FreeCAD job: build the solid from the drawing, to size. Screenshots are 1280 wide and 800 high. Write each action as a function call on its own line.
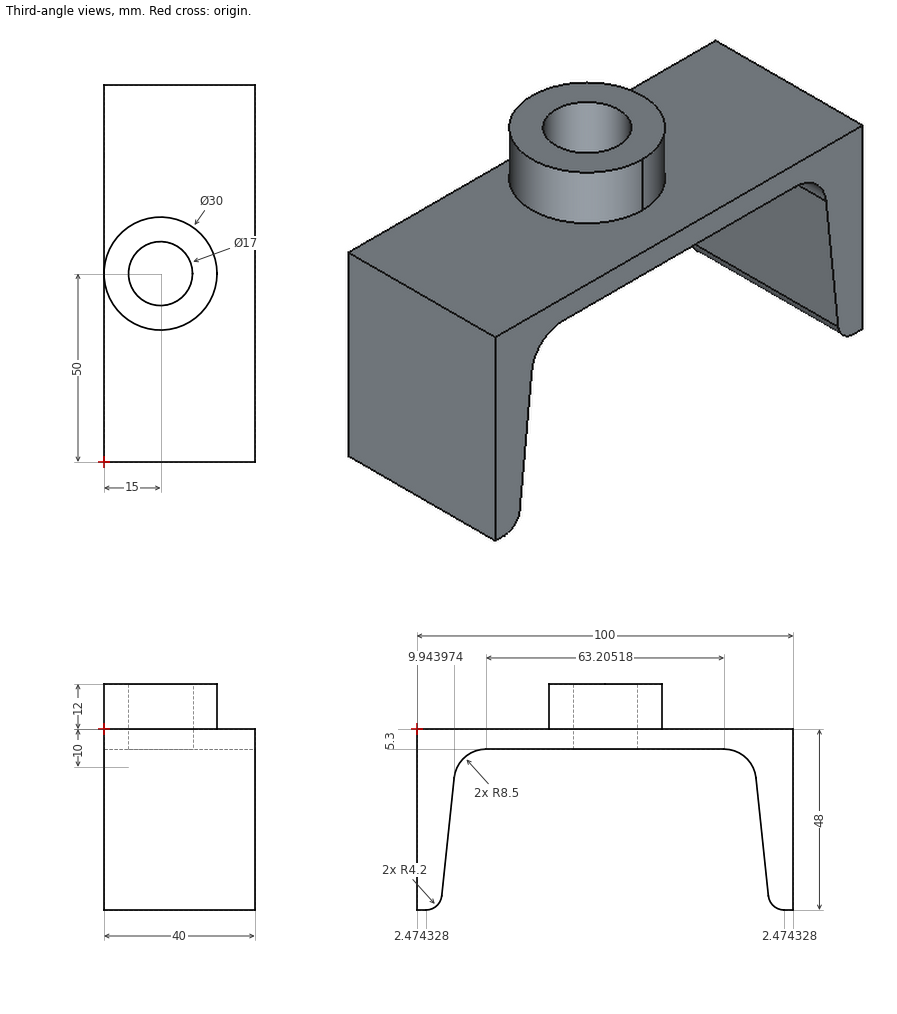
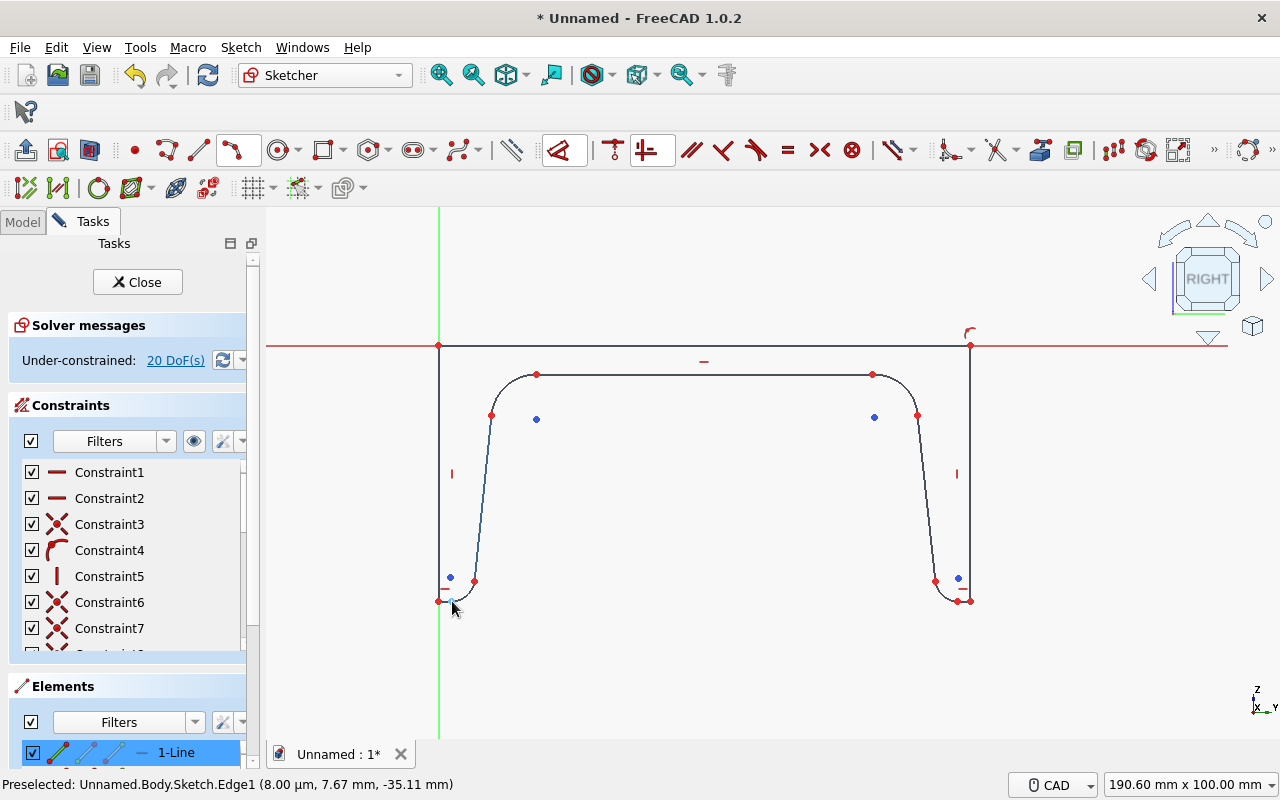
click(517, 379)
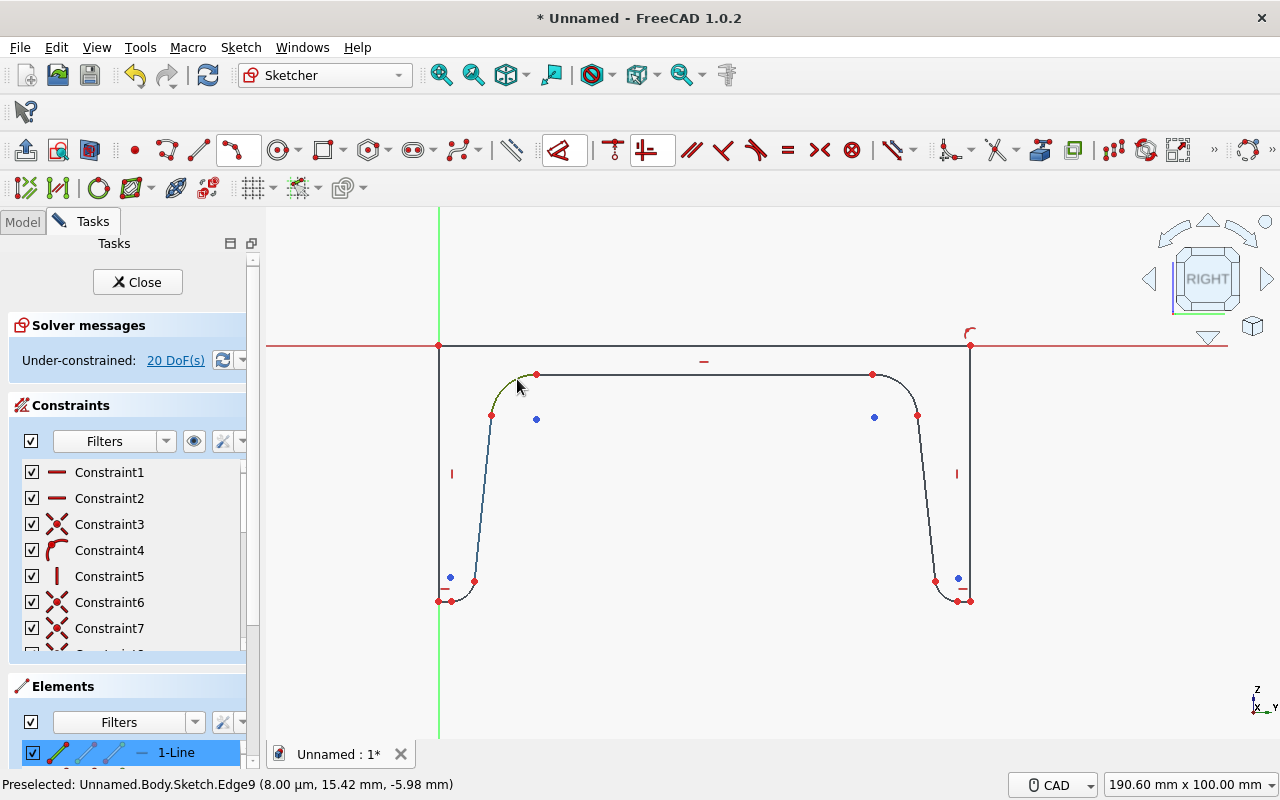
click(756, 150)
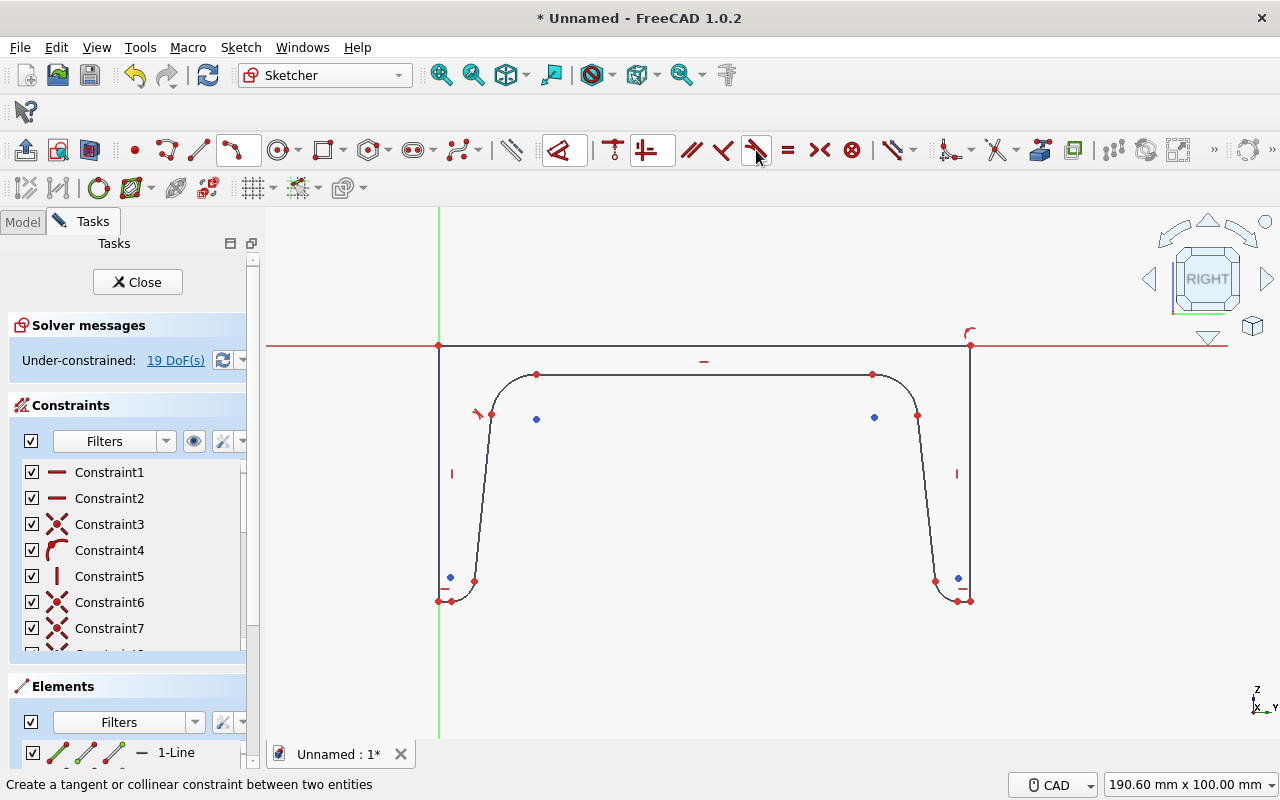
click(480, 532)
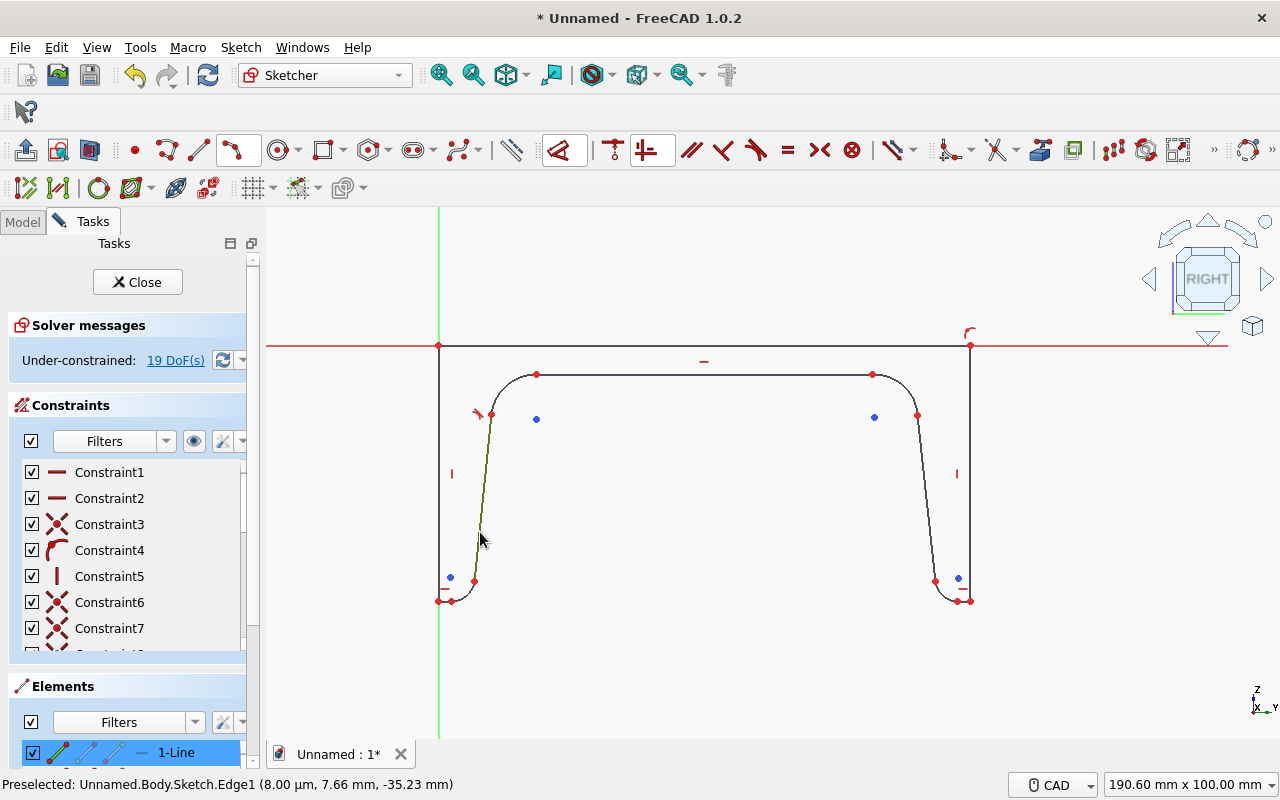
scroll(461, 599, up, 2)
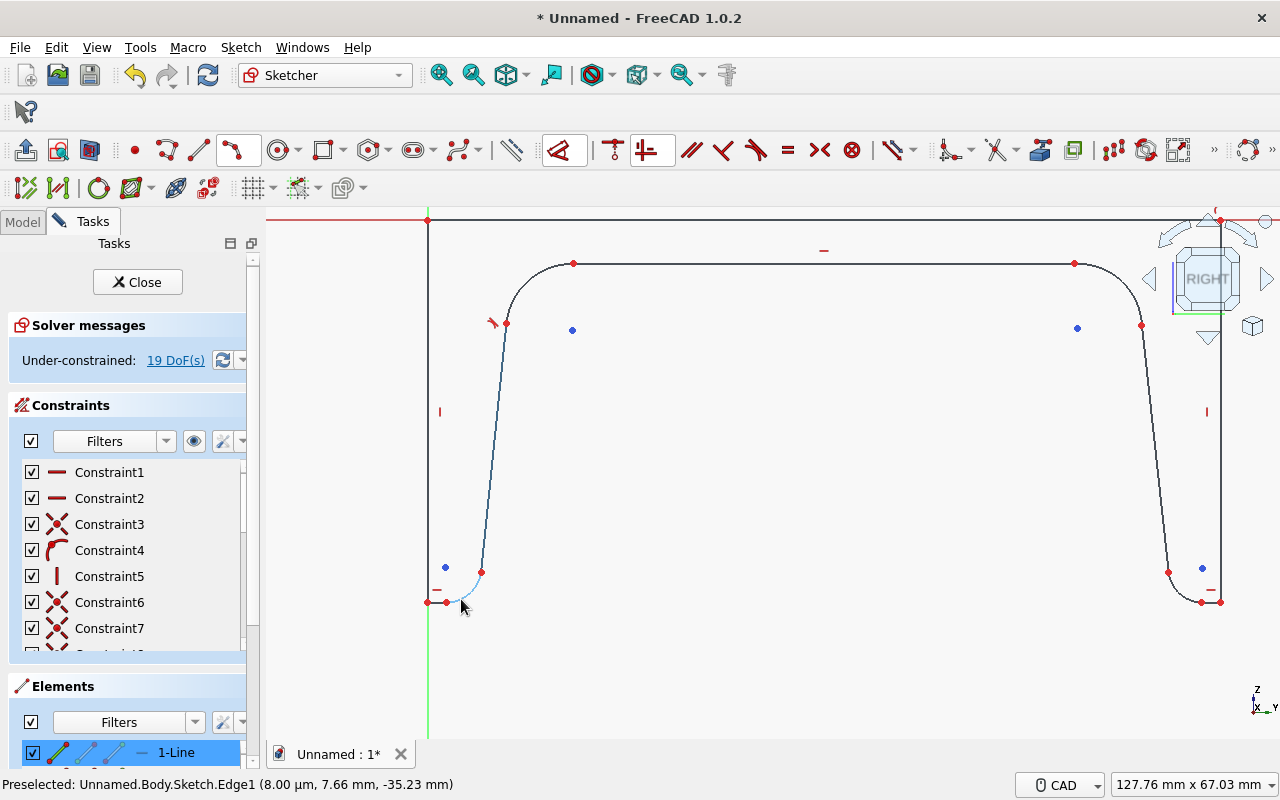
click(461, 599)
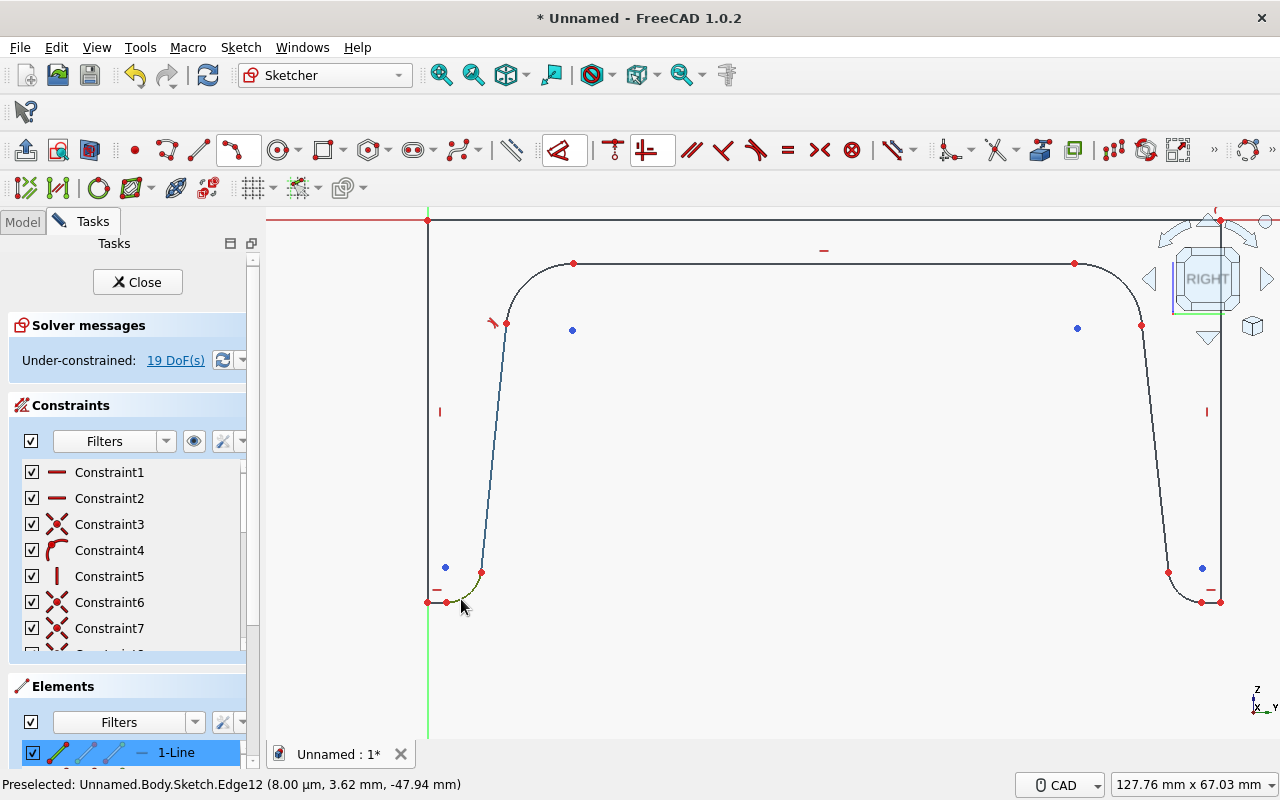
click(756, 150)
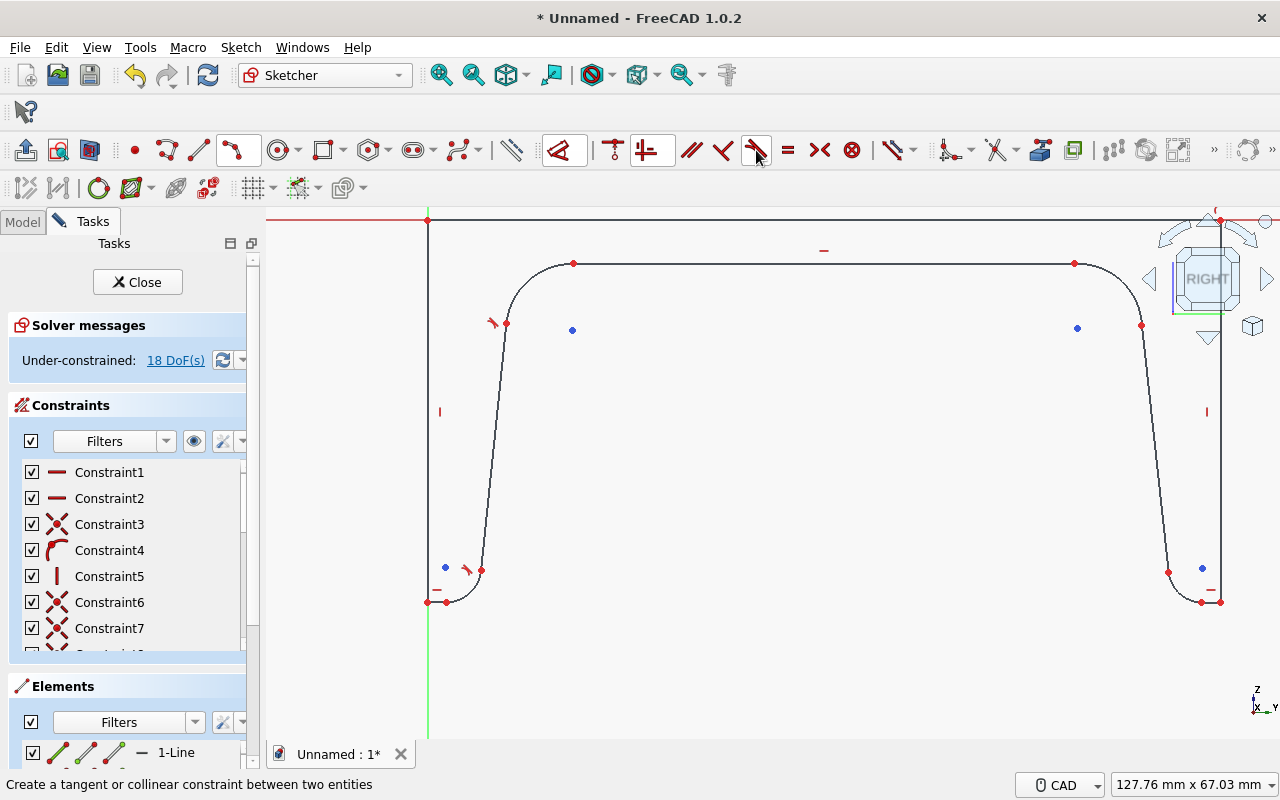
click(724, 264)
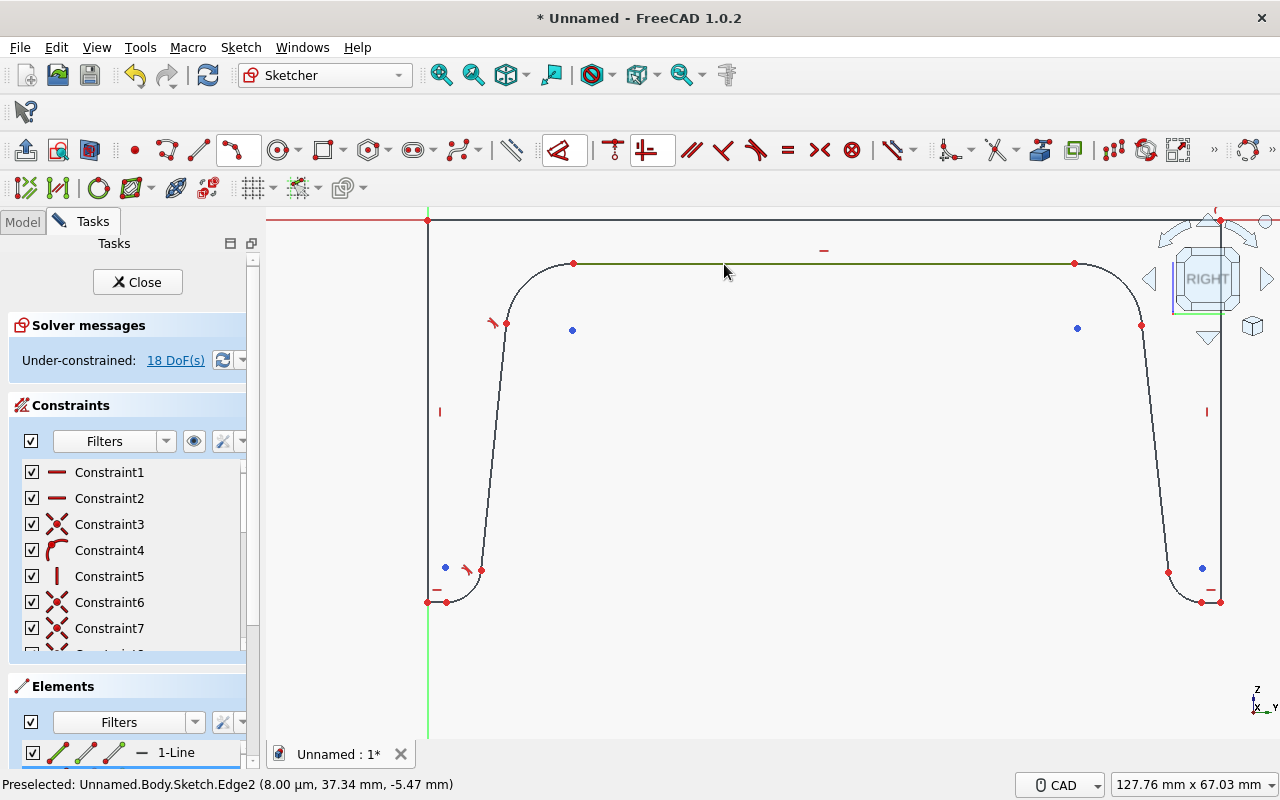
click(545, 270)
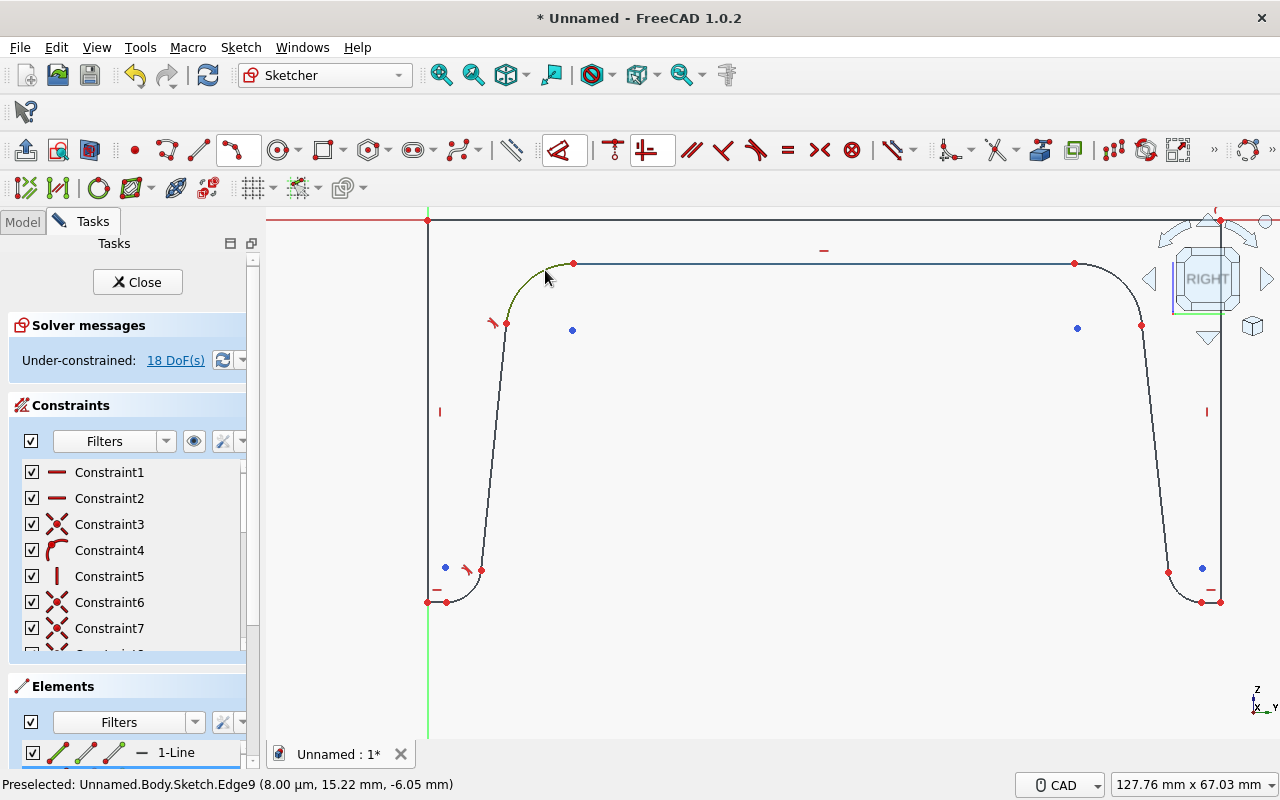
click(756, 150)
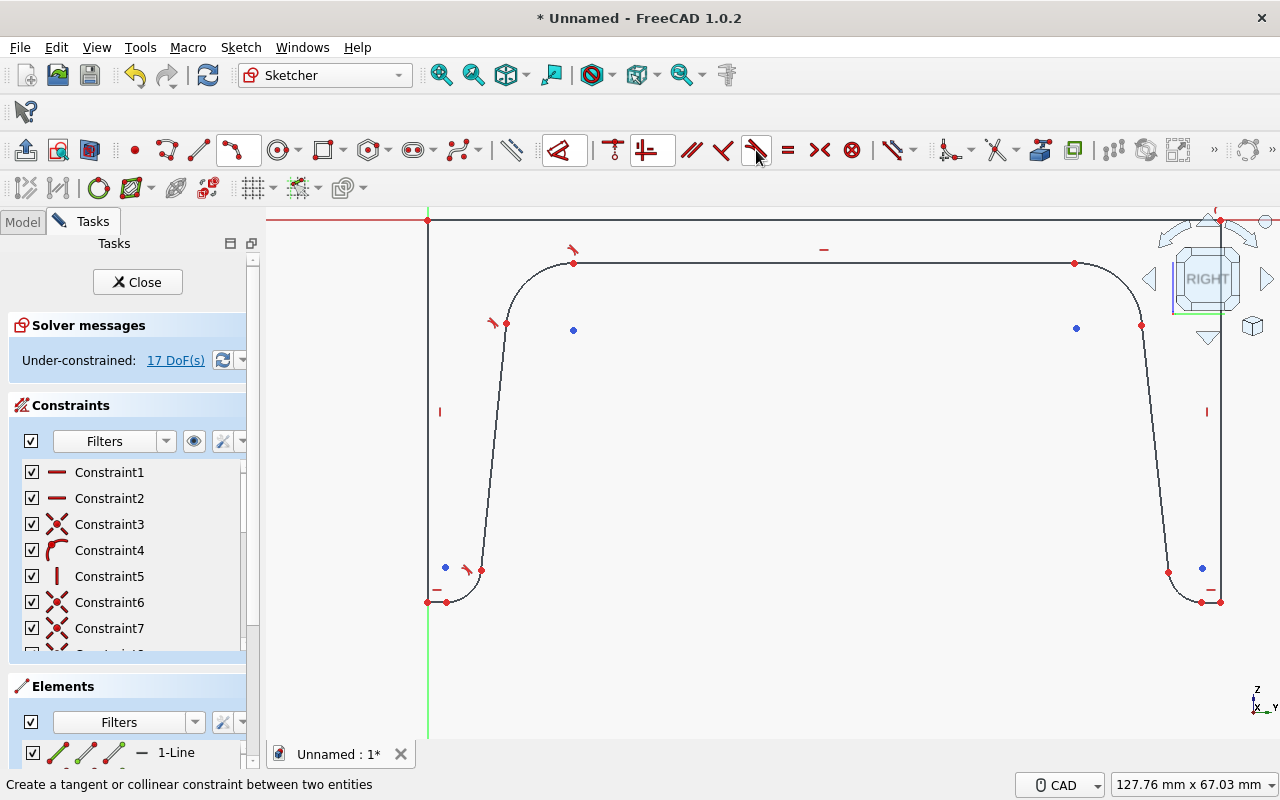
click(724, 263)